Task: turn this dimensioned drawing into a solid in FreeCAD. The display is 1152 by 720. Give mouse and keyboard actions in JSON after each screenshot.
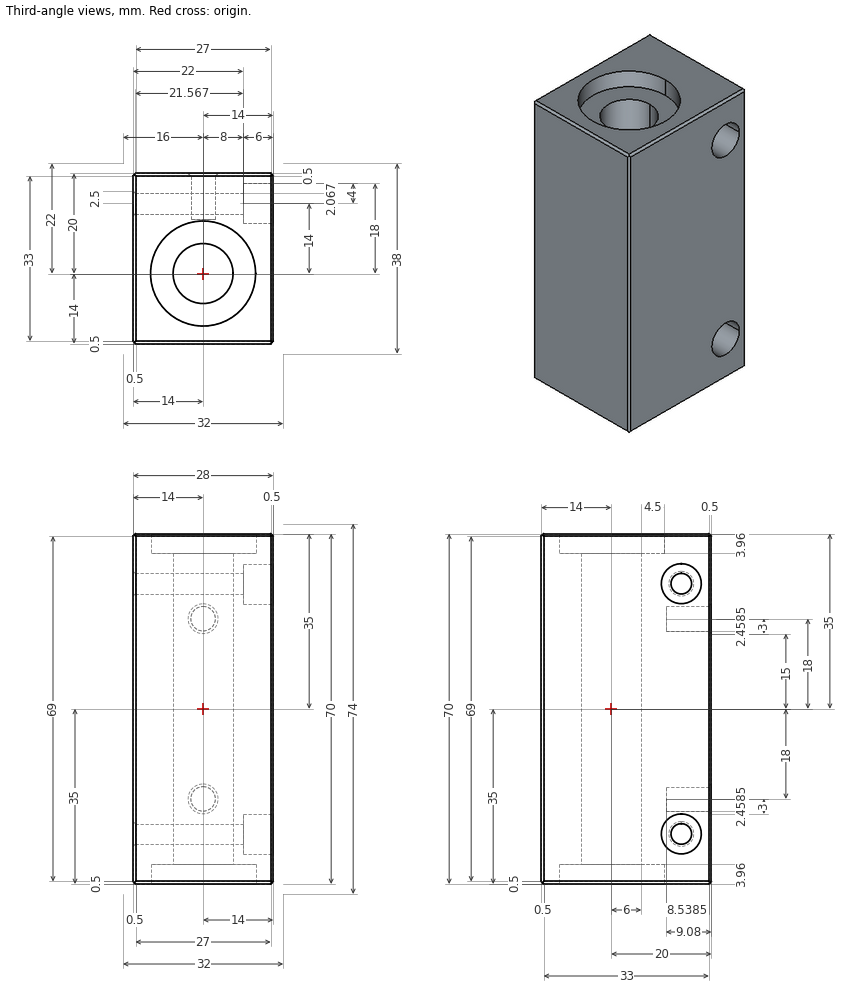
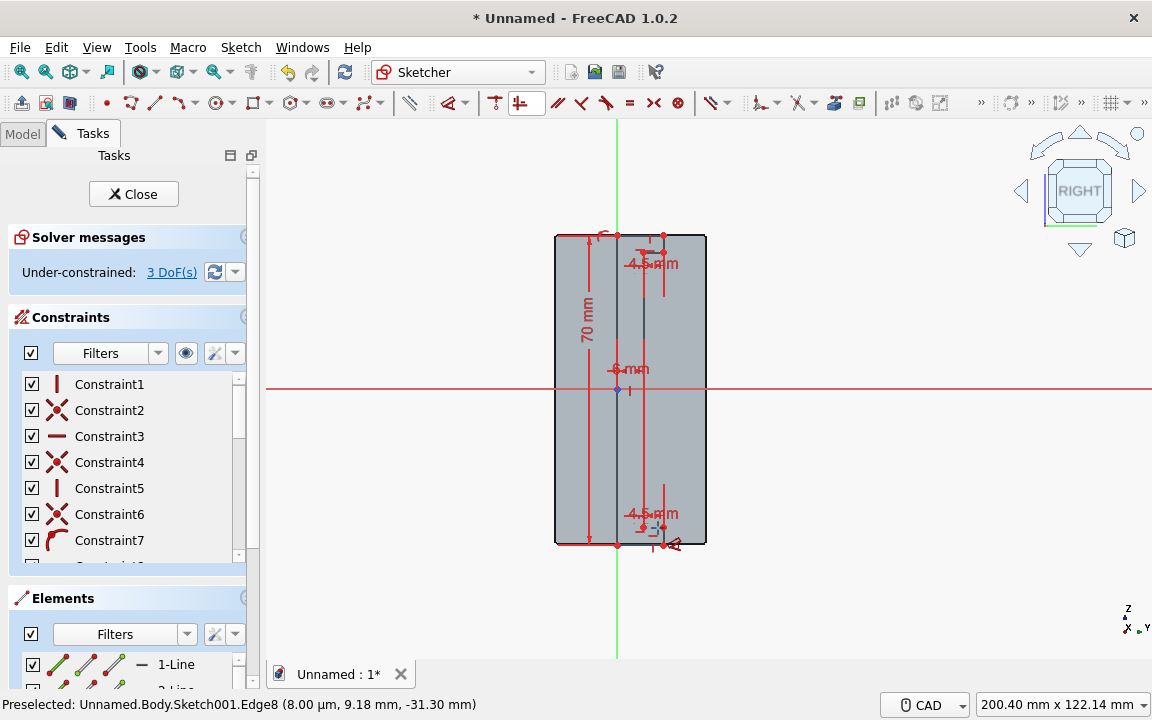
{"action": "left_click", "coordinate": [664, 236]}
{"action": "left_click", "coordinate": [698, 313]}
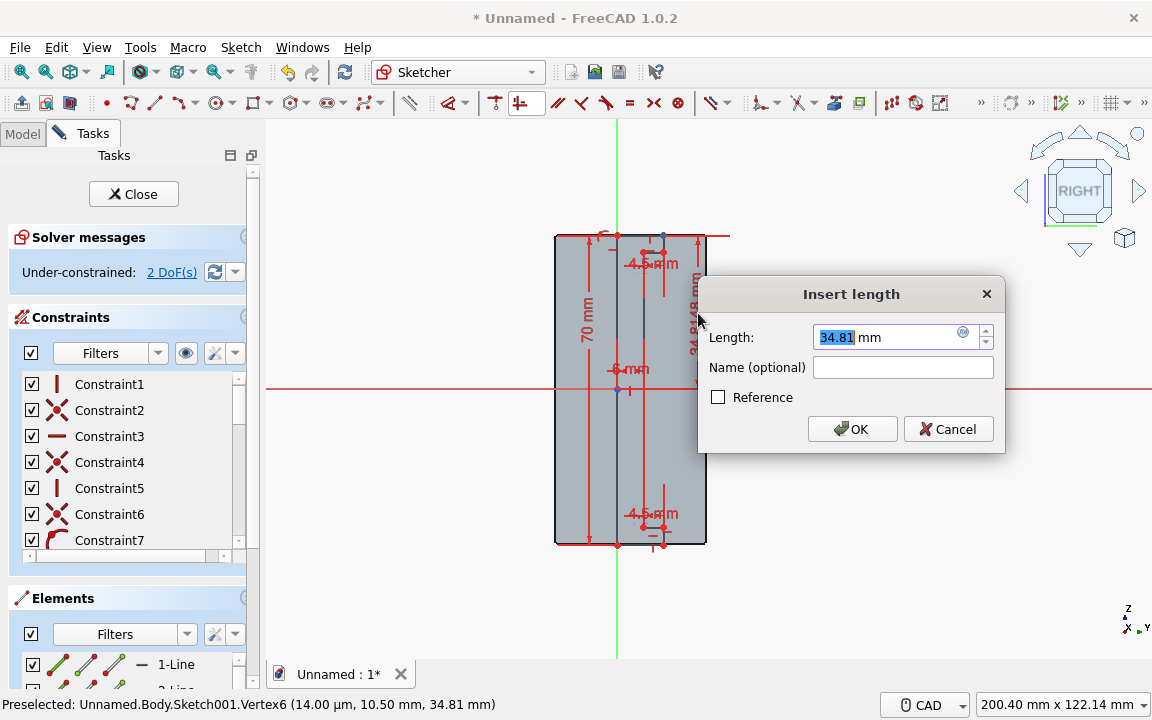
{"action": "type", "text": "35"}
{"action": "key", "text": "Return"}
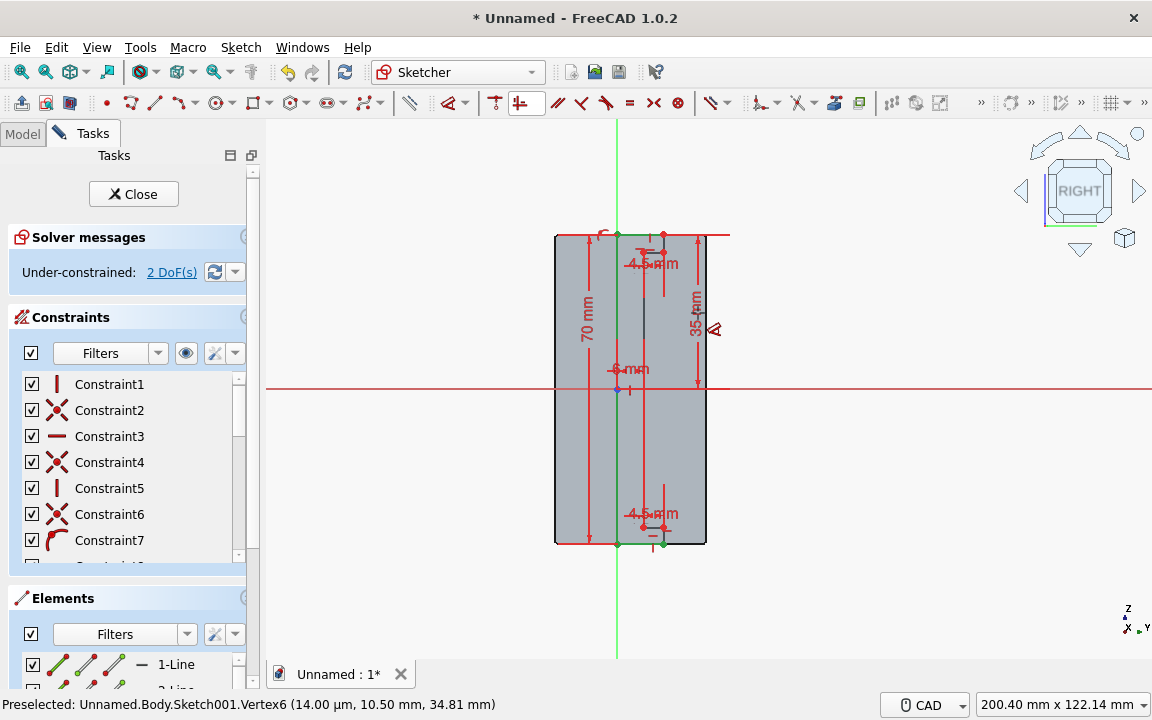
{"action": "scroll", "coordinate": [664, 244], "scroll_direction": "up", "scroll_amount": 5}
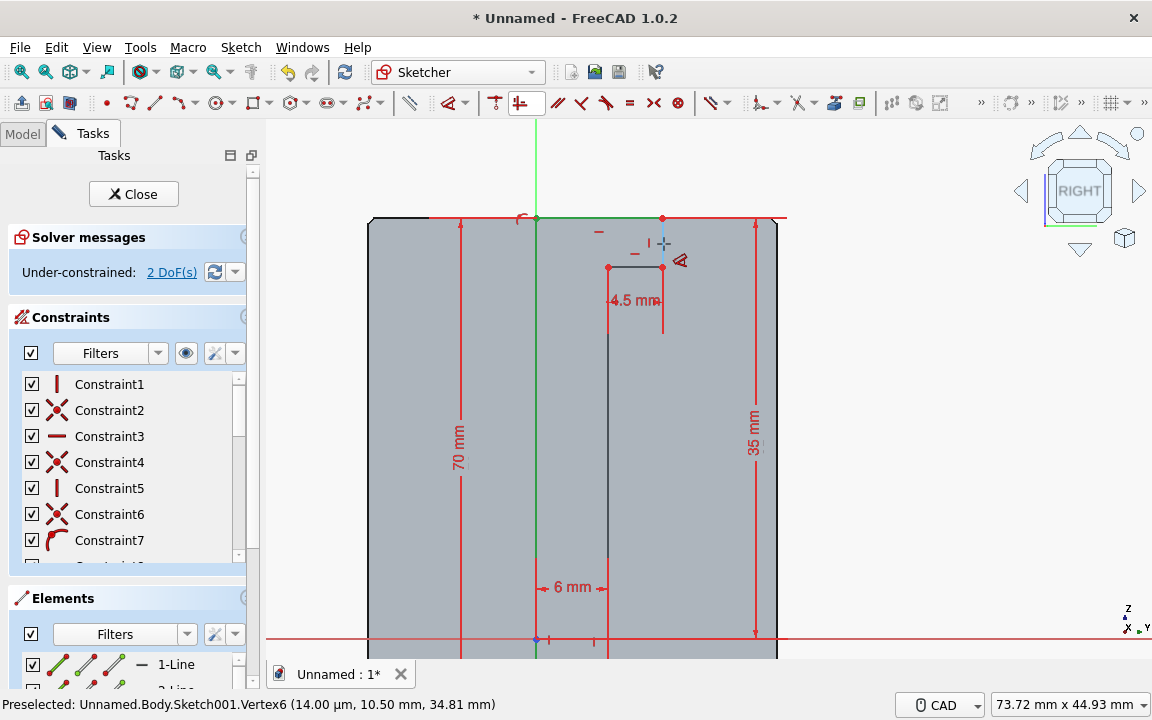
{"action": "left_click", "coordinate": [663, 243]}
{"action": "left_click", "coordinate": [697, 243]}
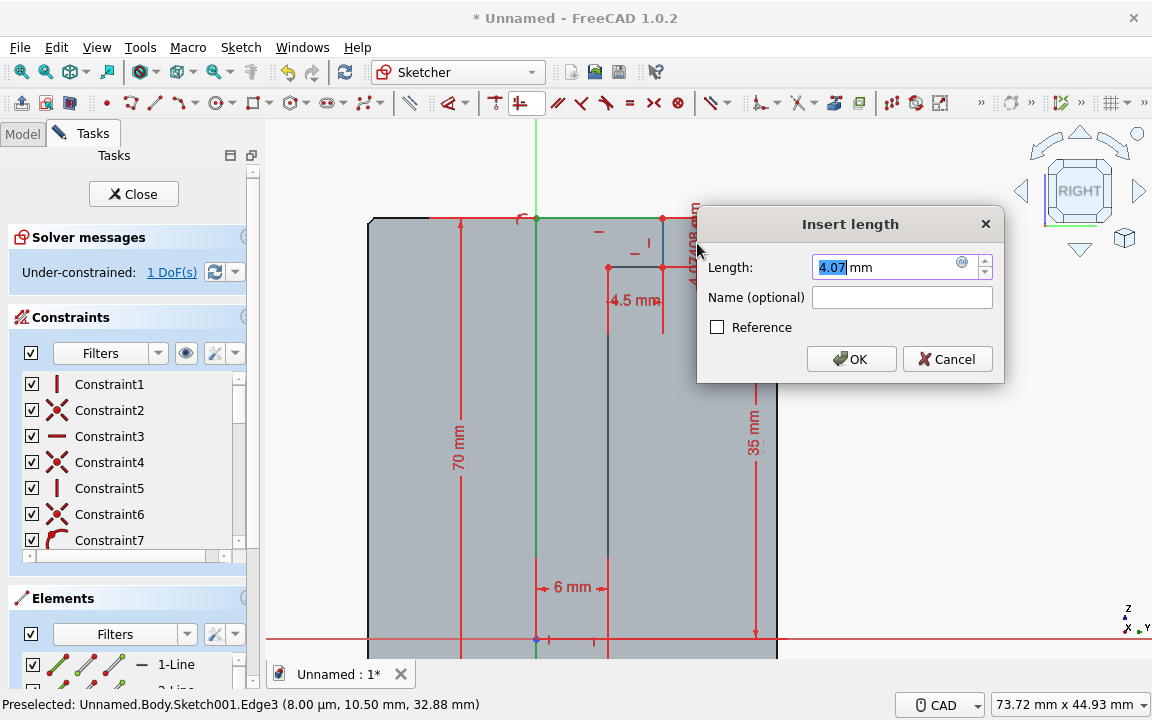
{"action": "type", "text": "3.96"}
{"action": "key", "text": "Return"}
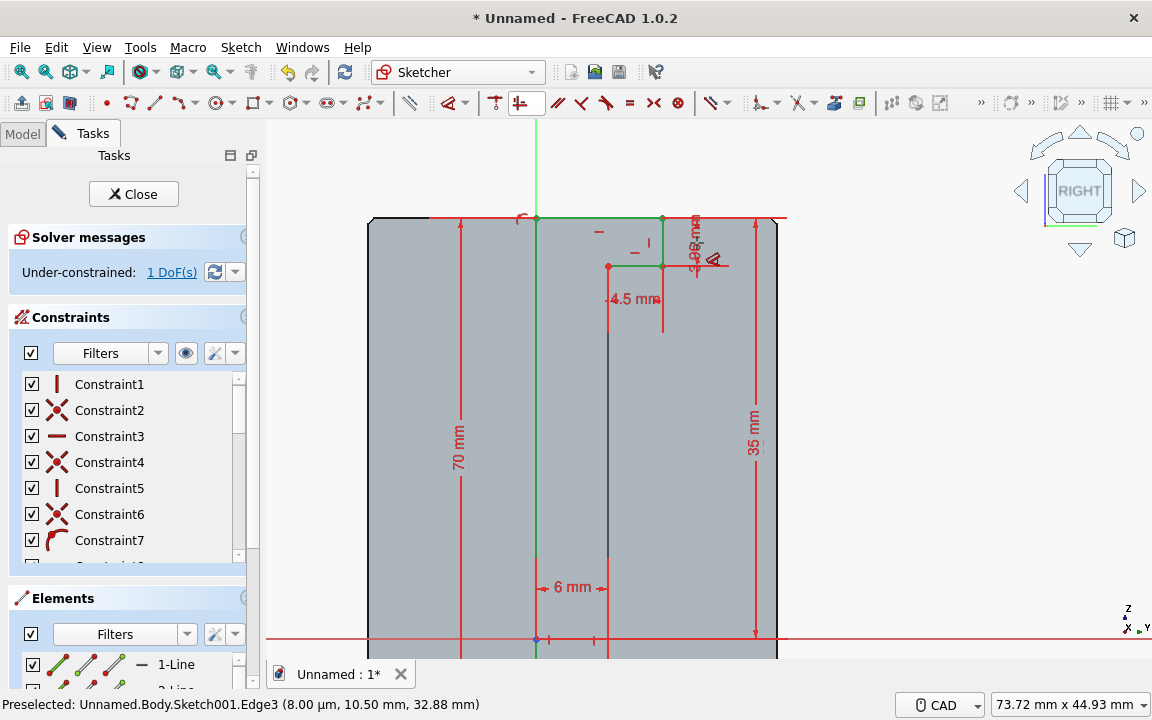
{"action": "scroll", "coordinate": [664, 243], "scroll_direction": "down", "scroll_amount": 5}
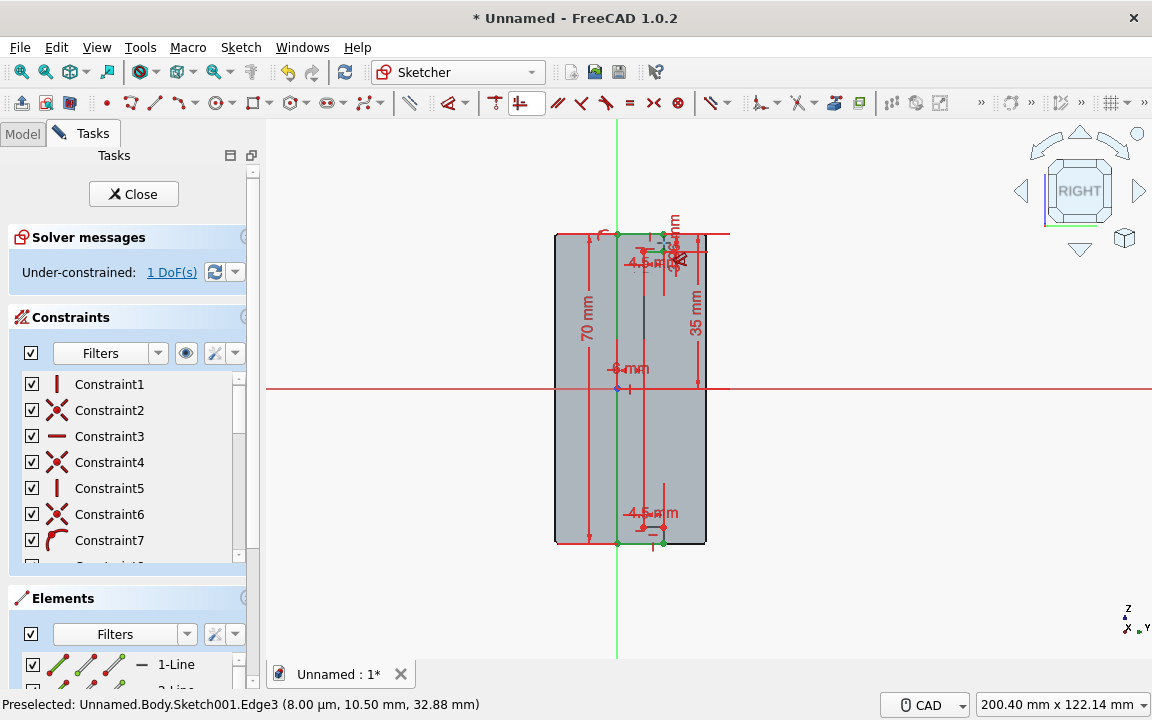
{"action": "scroll", "coordinate": [664, 539], "scroll_direction": "up", "scroll_amount": 6}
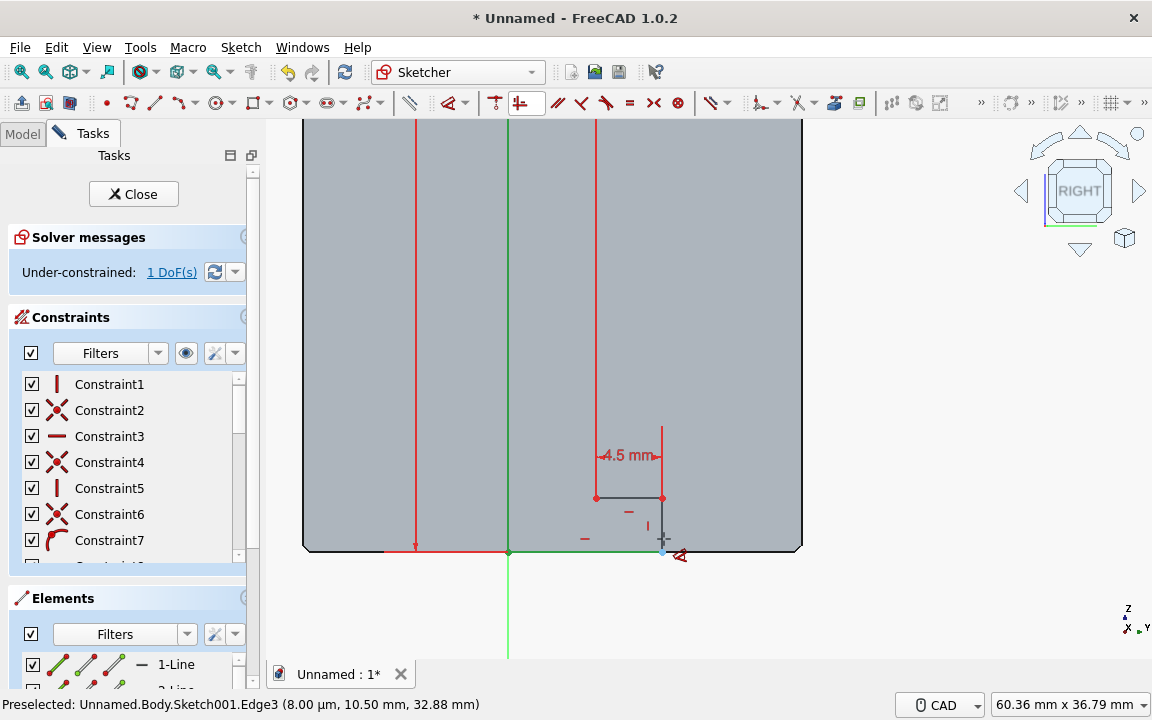
{"action": "left_click", "coordinate": [662, 536]}
{"action": "left_click", "coordinate": [696, 525]}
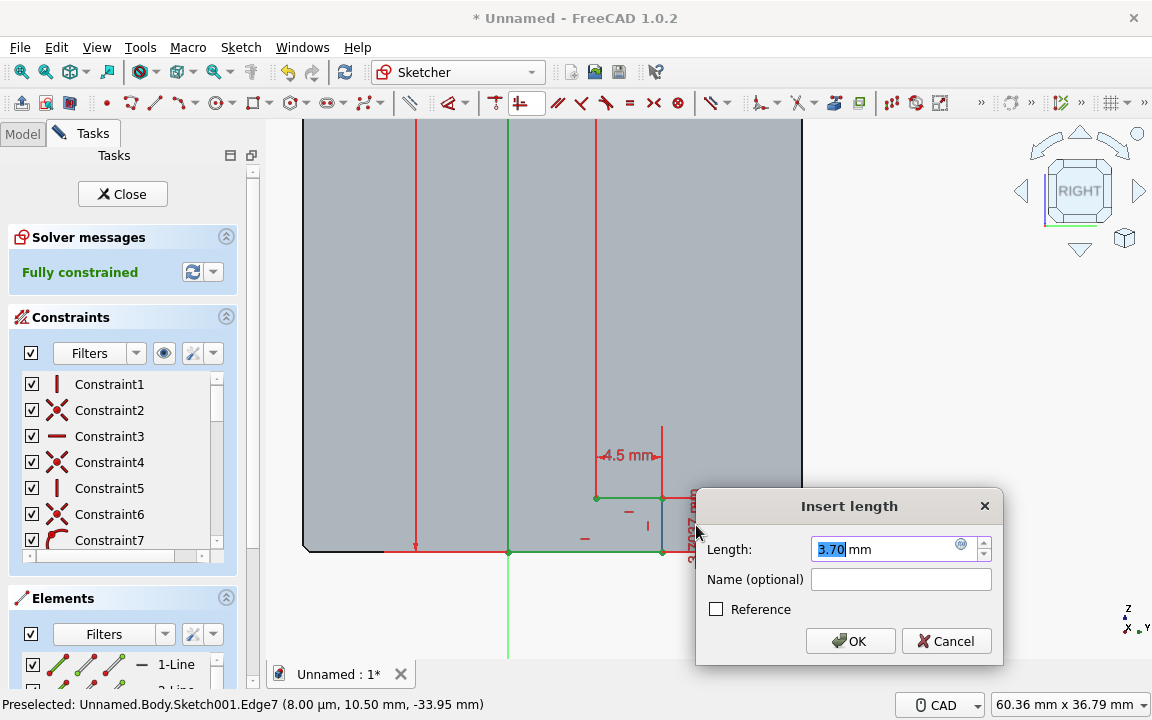
{"action": "type", "text": "3.96"}
{"action": "key", "text": "Return"}
{"action": "key", "text": "Escape"}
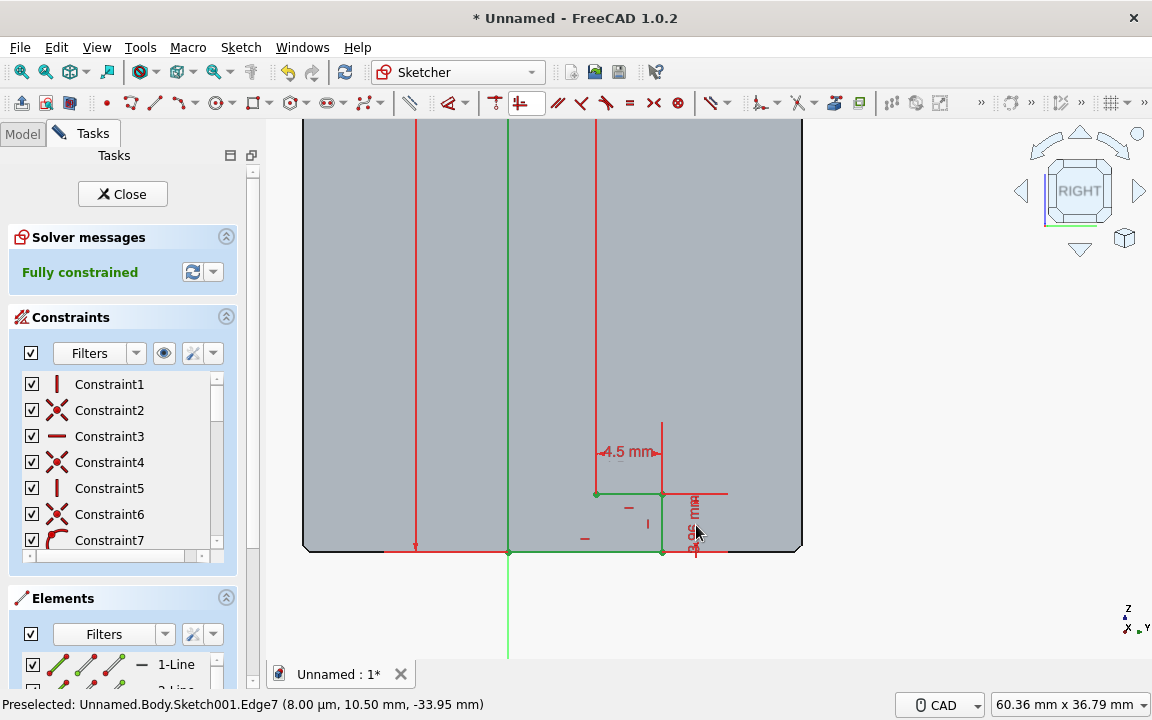
{"action": "left_click", "coordinate": [123, 194]}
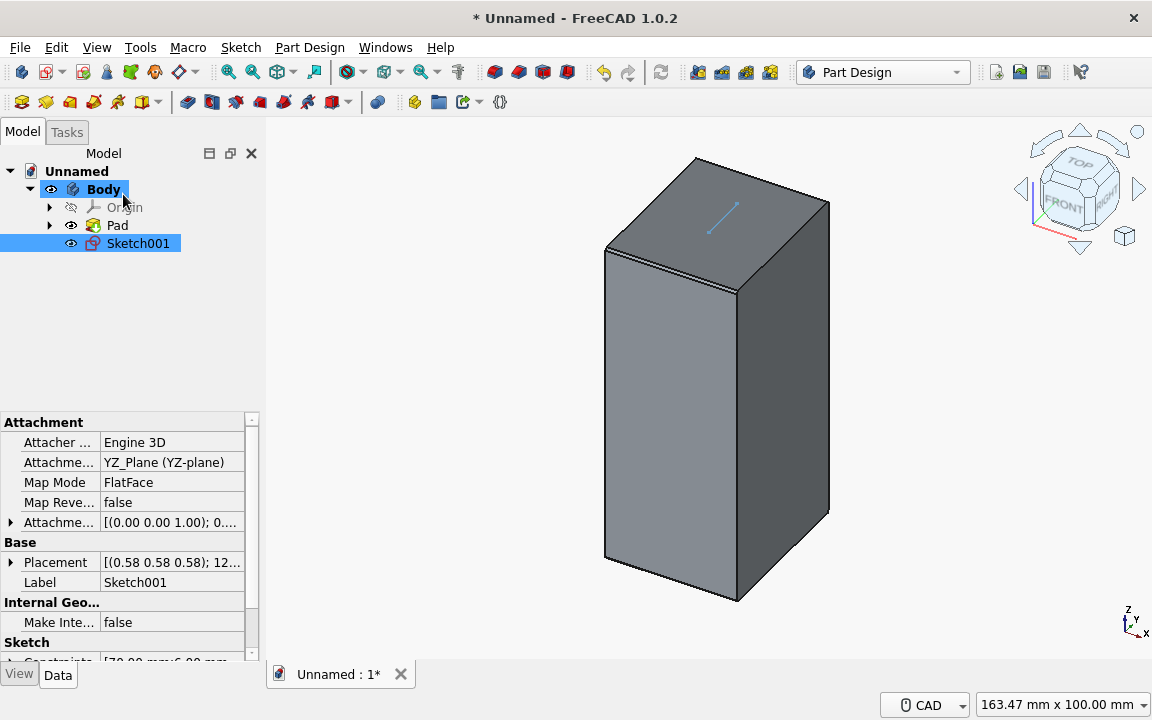
{"action": "left_click", "coordinate": [236, 102]}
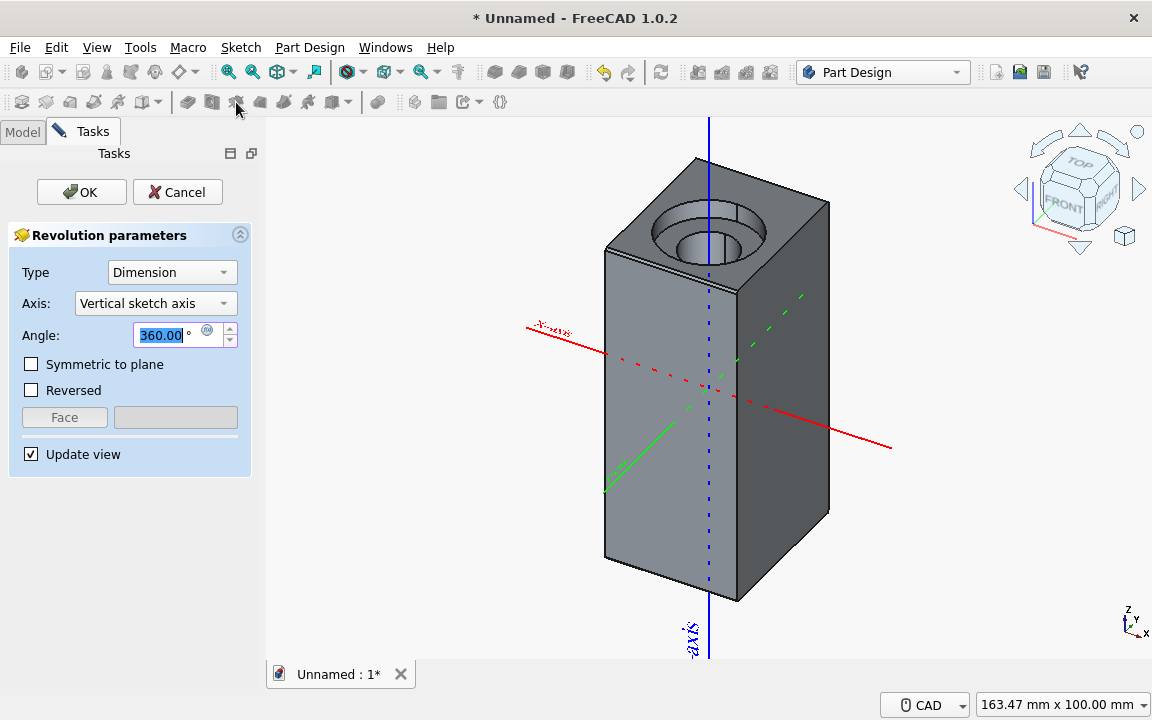
{"action": "left_click", "coordinate": [82, 192]}